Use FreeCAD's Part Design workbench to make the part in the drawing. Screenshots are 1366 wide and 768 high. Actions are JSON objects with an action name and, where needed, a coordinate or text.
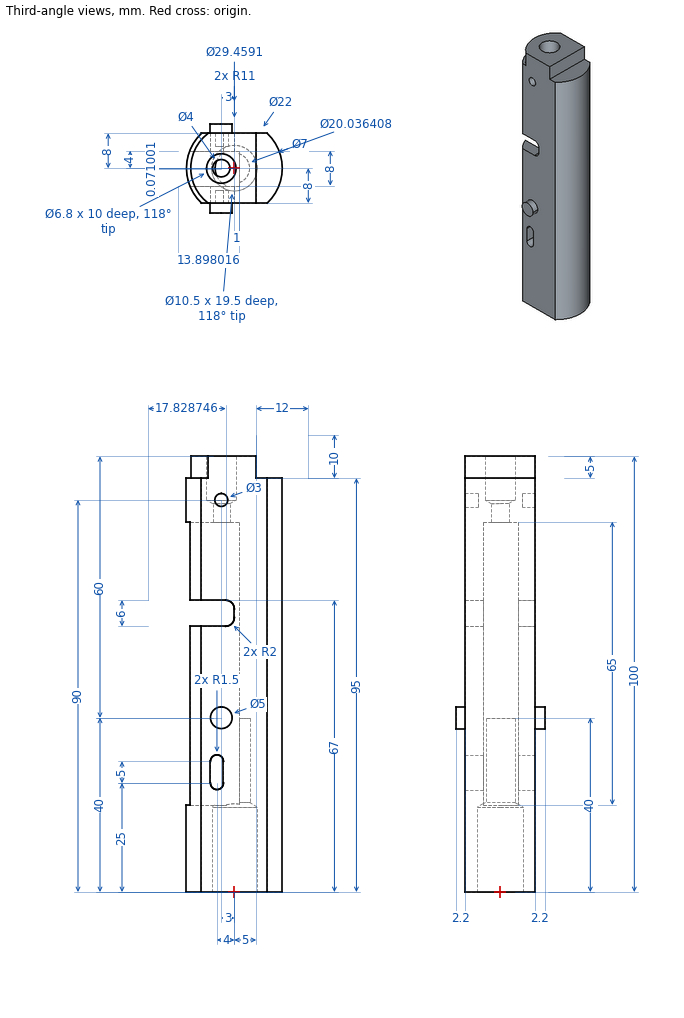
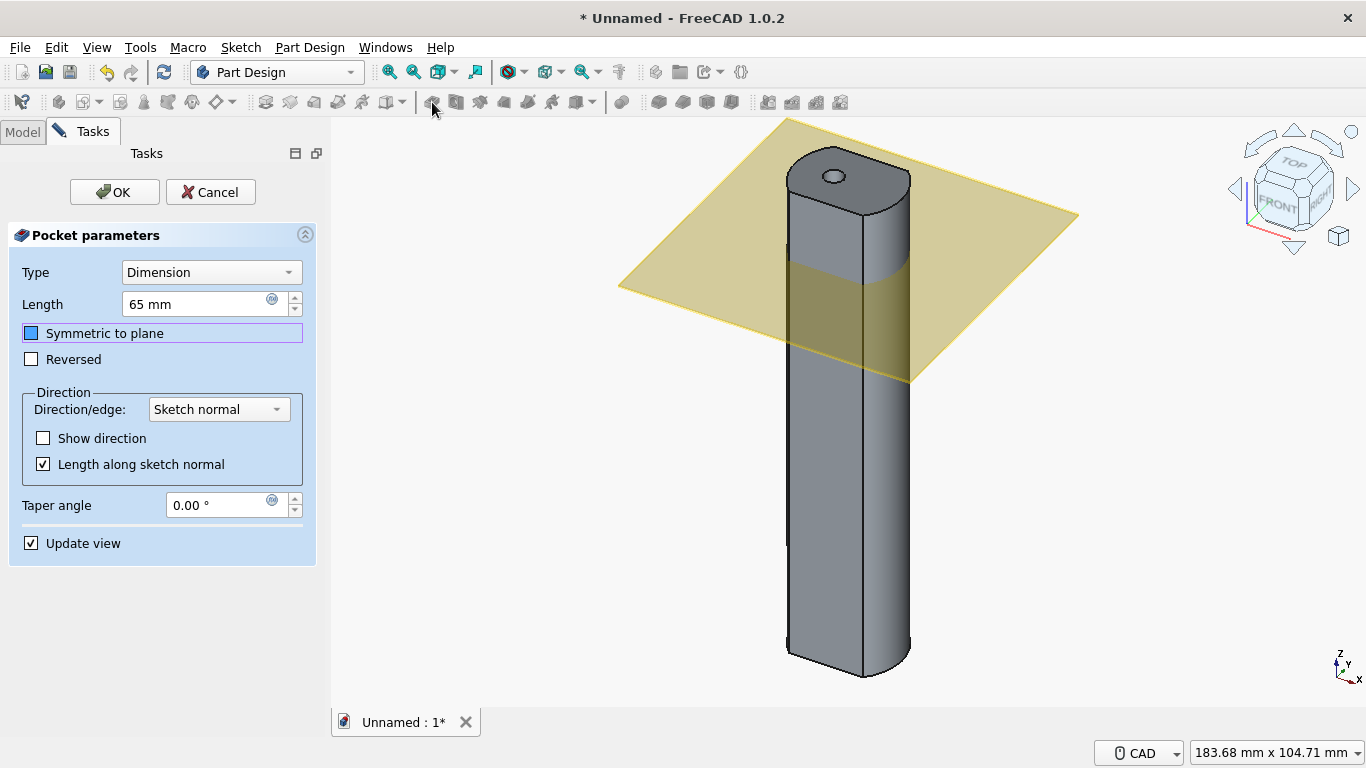
{"action": "left_click", "coordinate": [115, 192]}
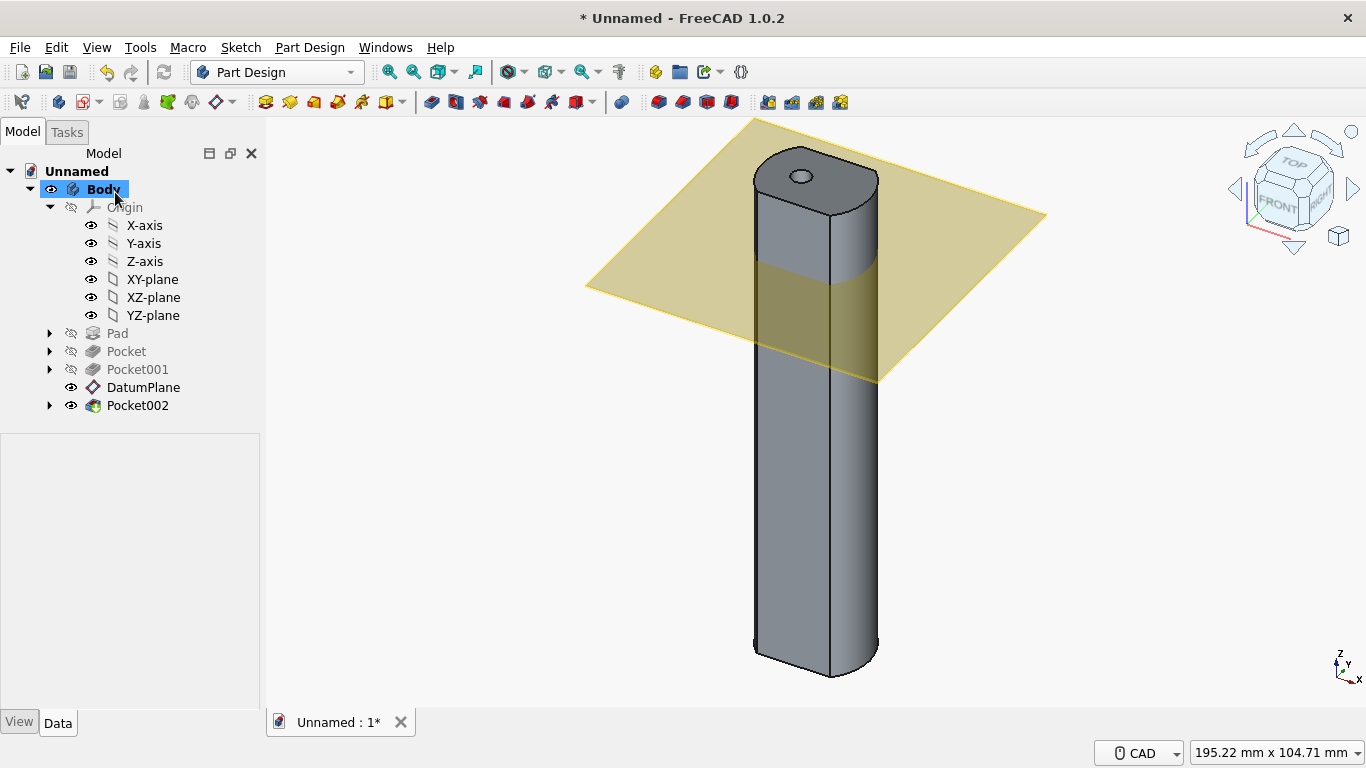
{"action": "left_click", "coordinate": [116, 387]}
{"action": "key", "text": "space"}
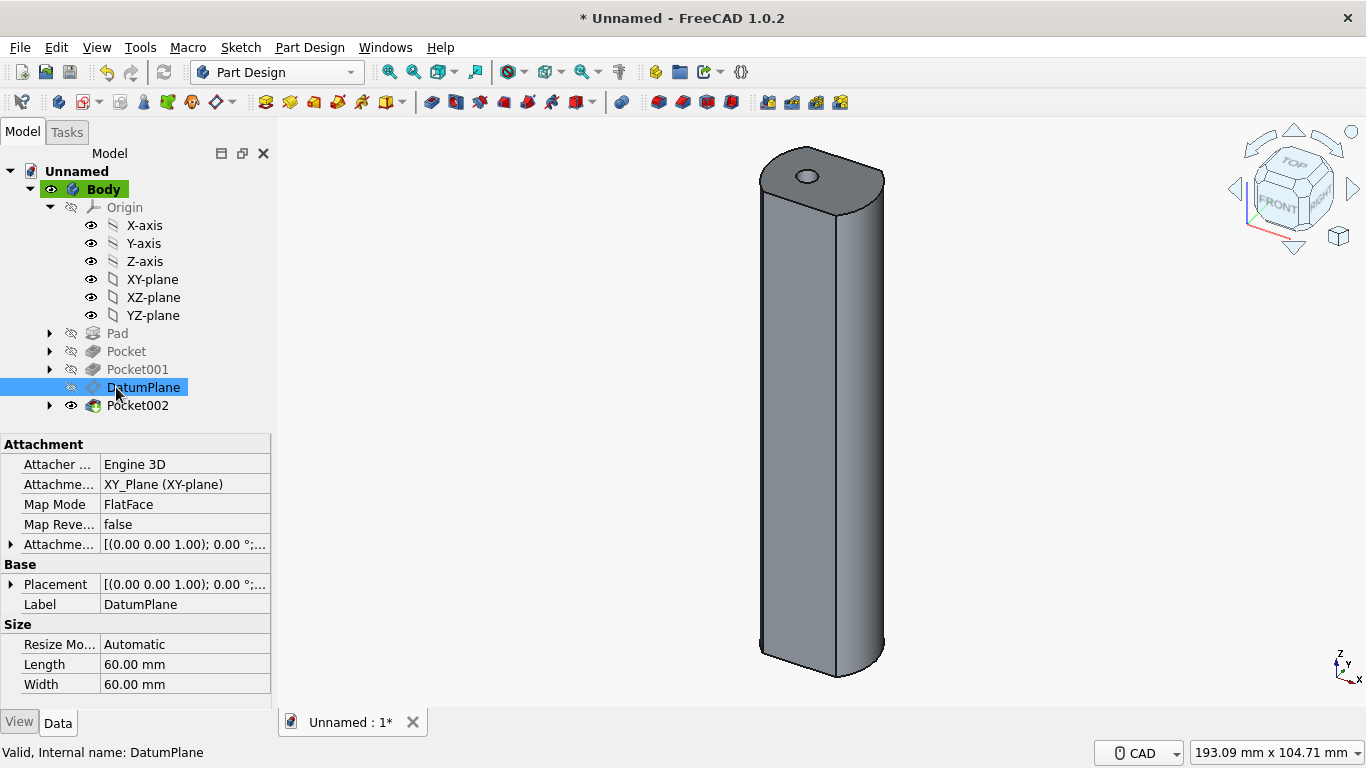
{"action": "left_click", "coordinate": [799, 302]}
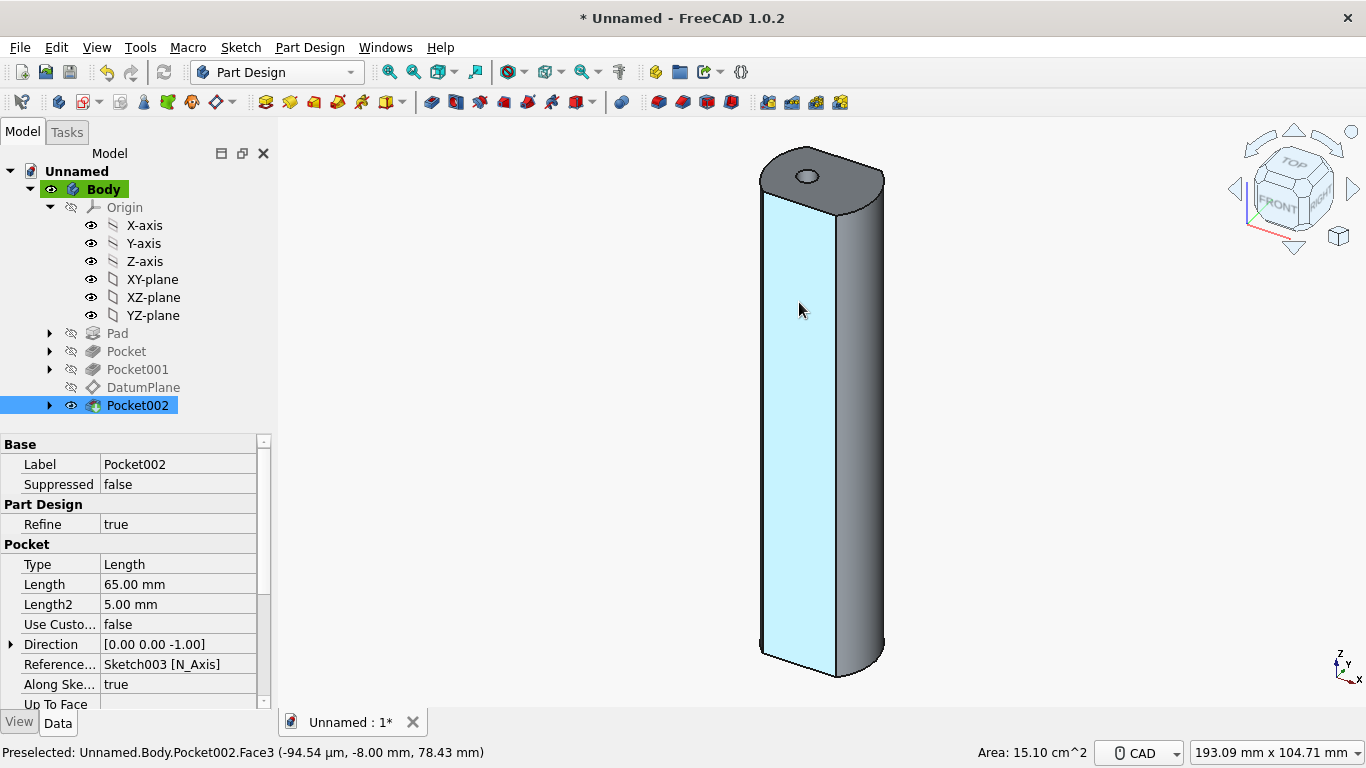
{"action": "left_click", "coordinate": [84, 102]}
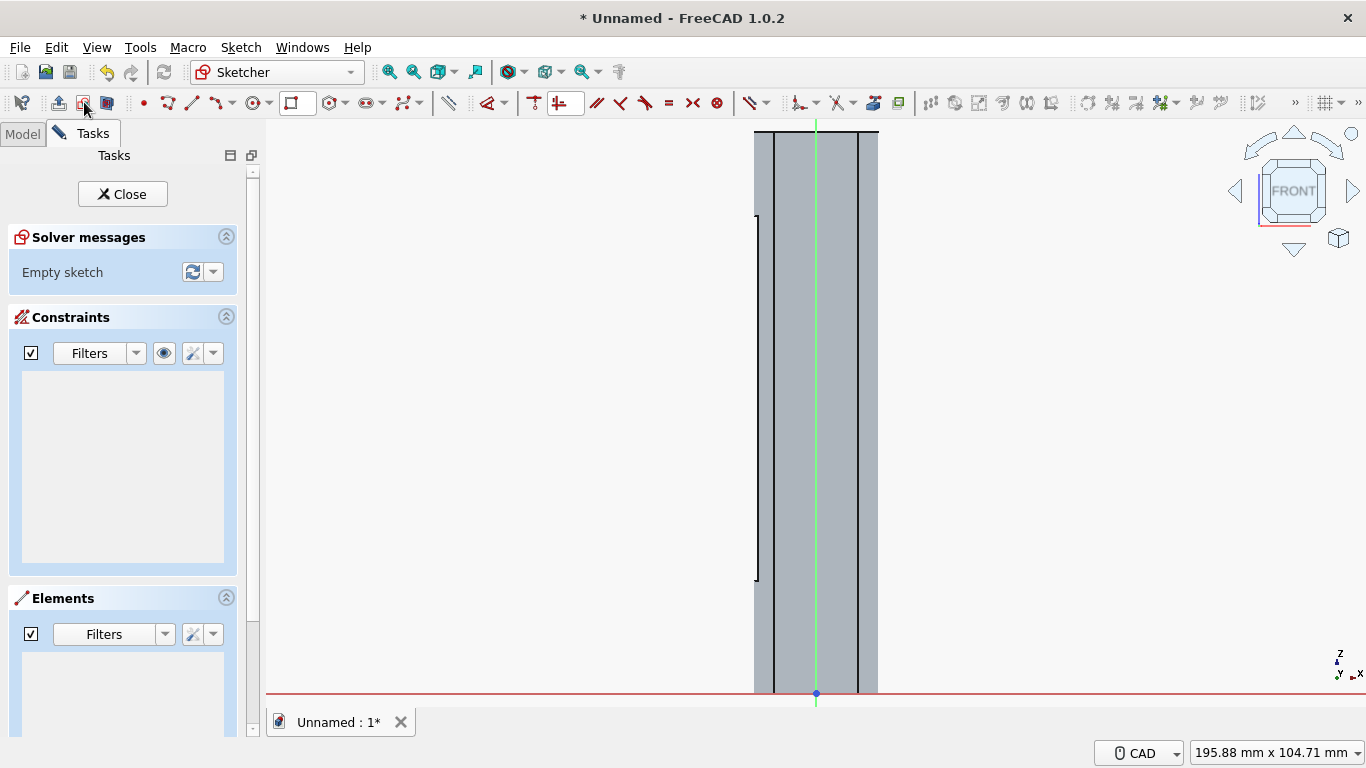
{"action": "scroll", "coordinate": [748, 413], "scroll_direction": "down", "scroll_amount": 5}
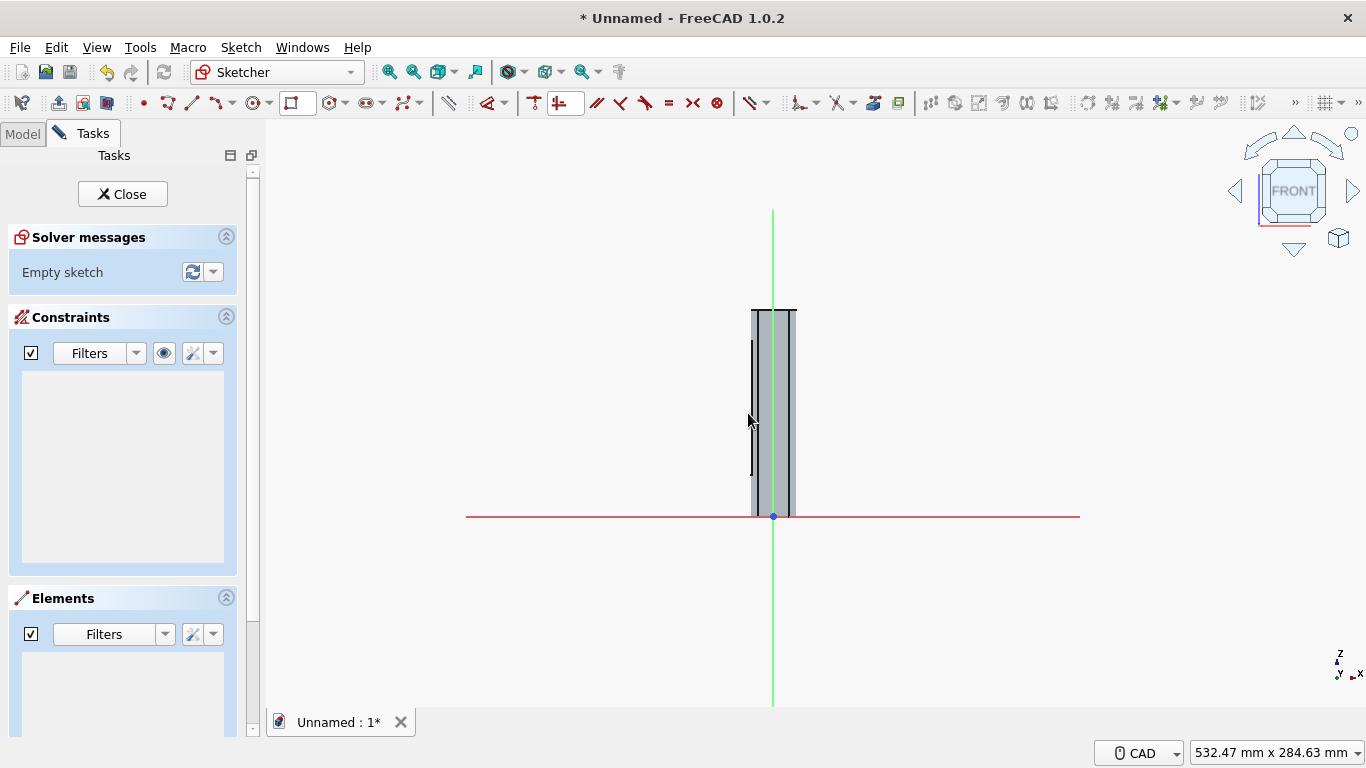
{"action": "scroll", "coordinate": [799, 305], "scroll_direction": "up", "scroll_amount": 15}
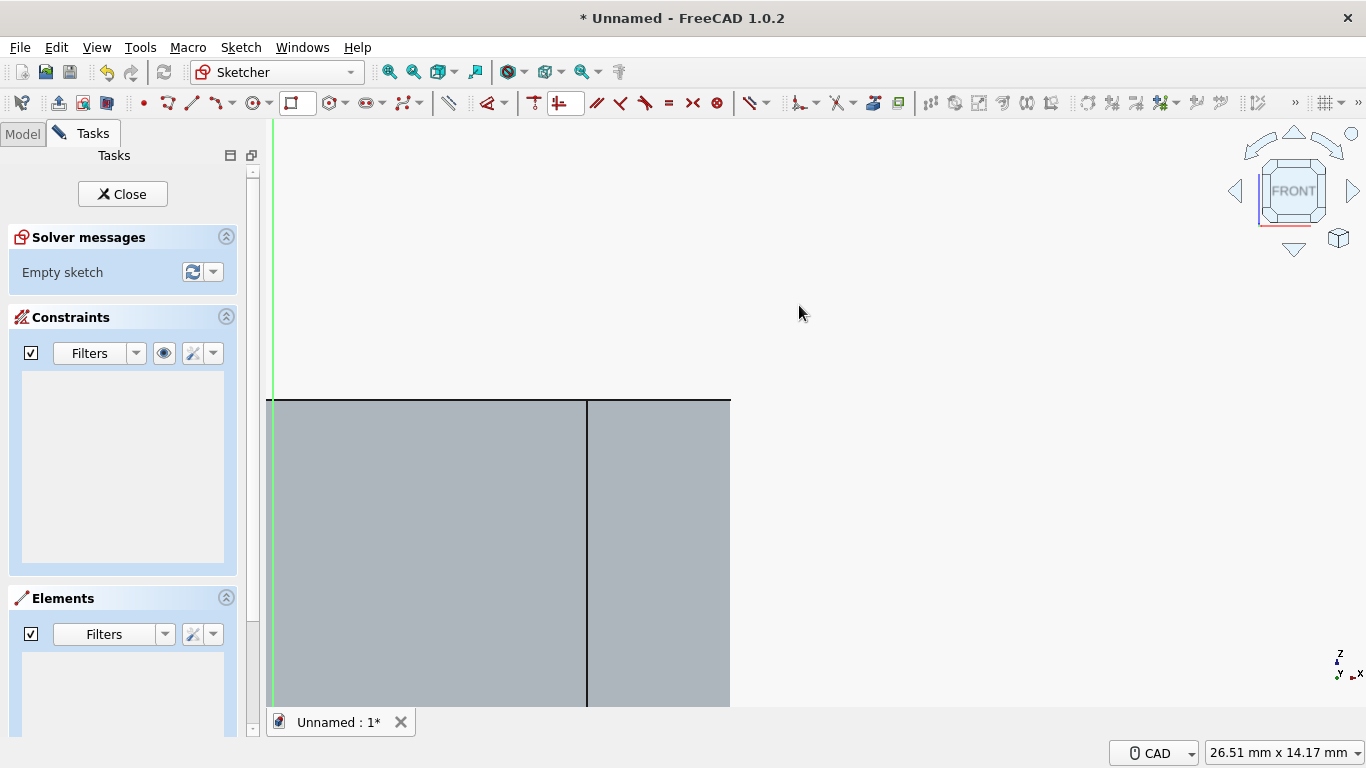
{"action": "left_click", "coordinate": [292, 104]}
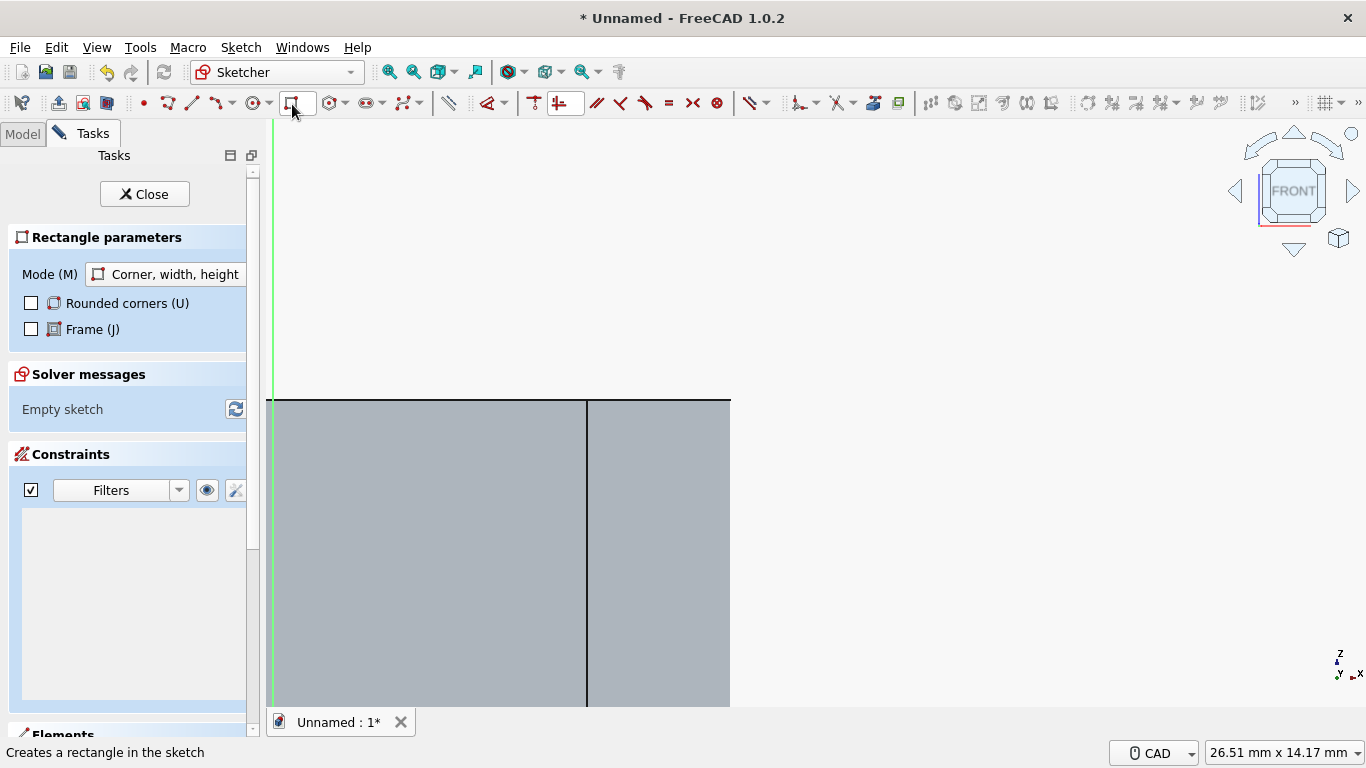
{"action": "left_click", "coordinate": [481, 192]}
{"action": "mouse_move", "coordinate": [979, 607]}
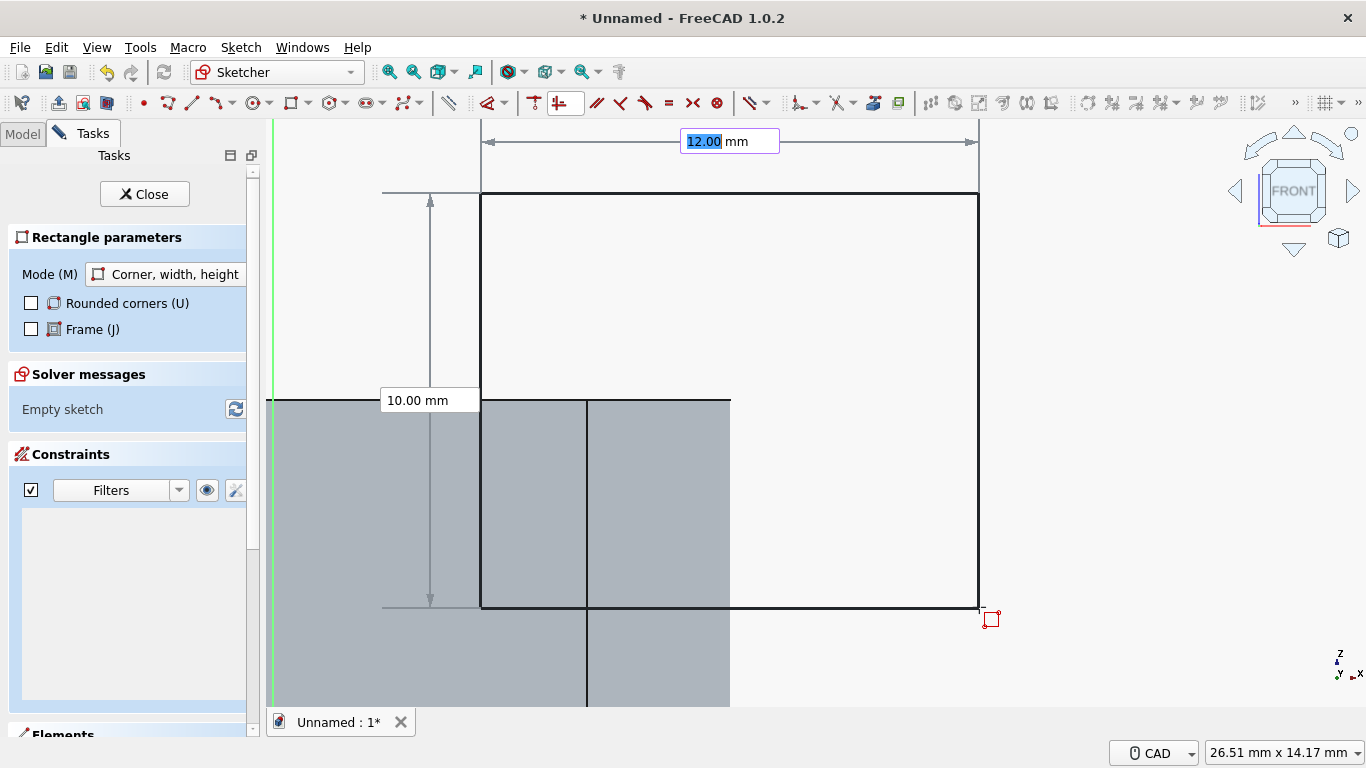
{"action": "type", "text": "12"}
{"action": "key", "text": "Tab"}
{"action": "type", "text": "10"}
{"action": "key", "text": "Return"}
{"action": "key", "text": "Escape"}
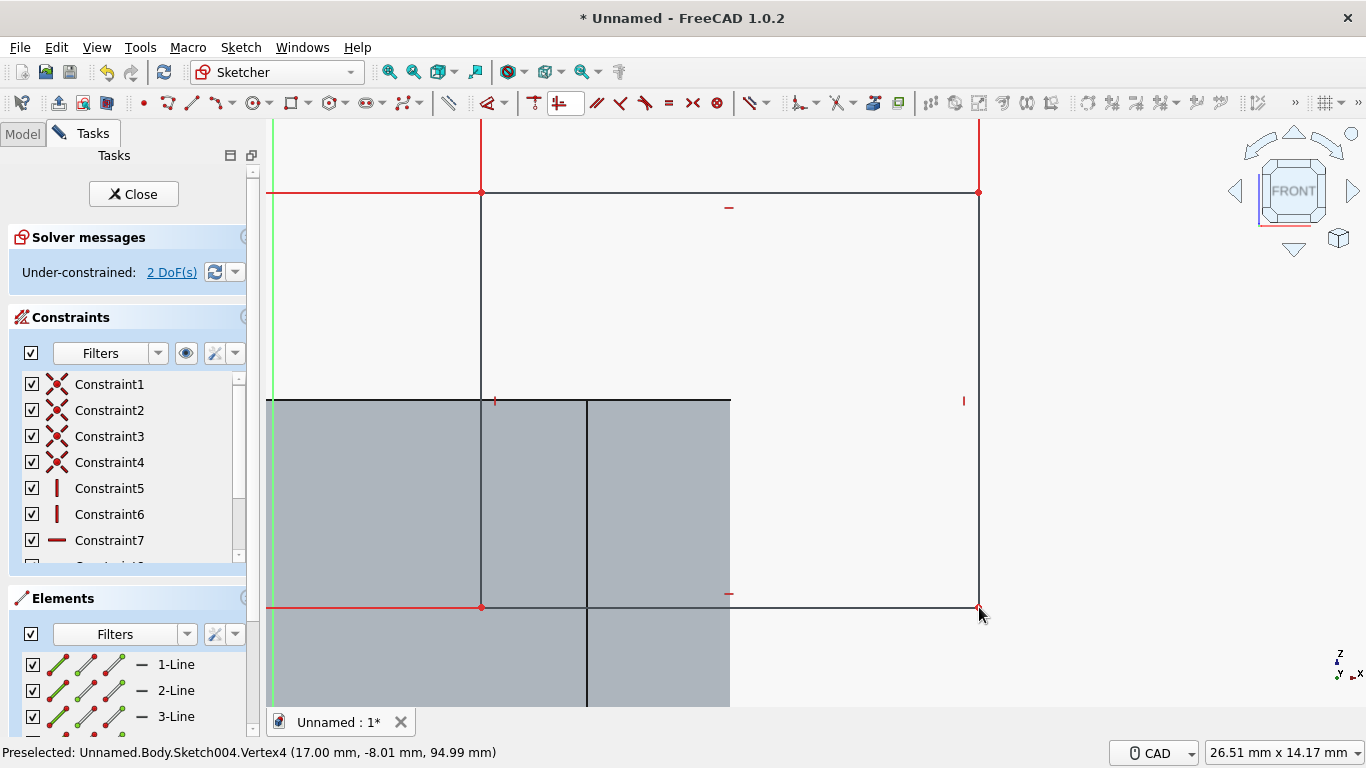
{"action": "key", "text": "d"}